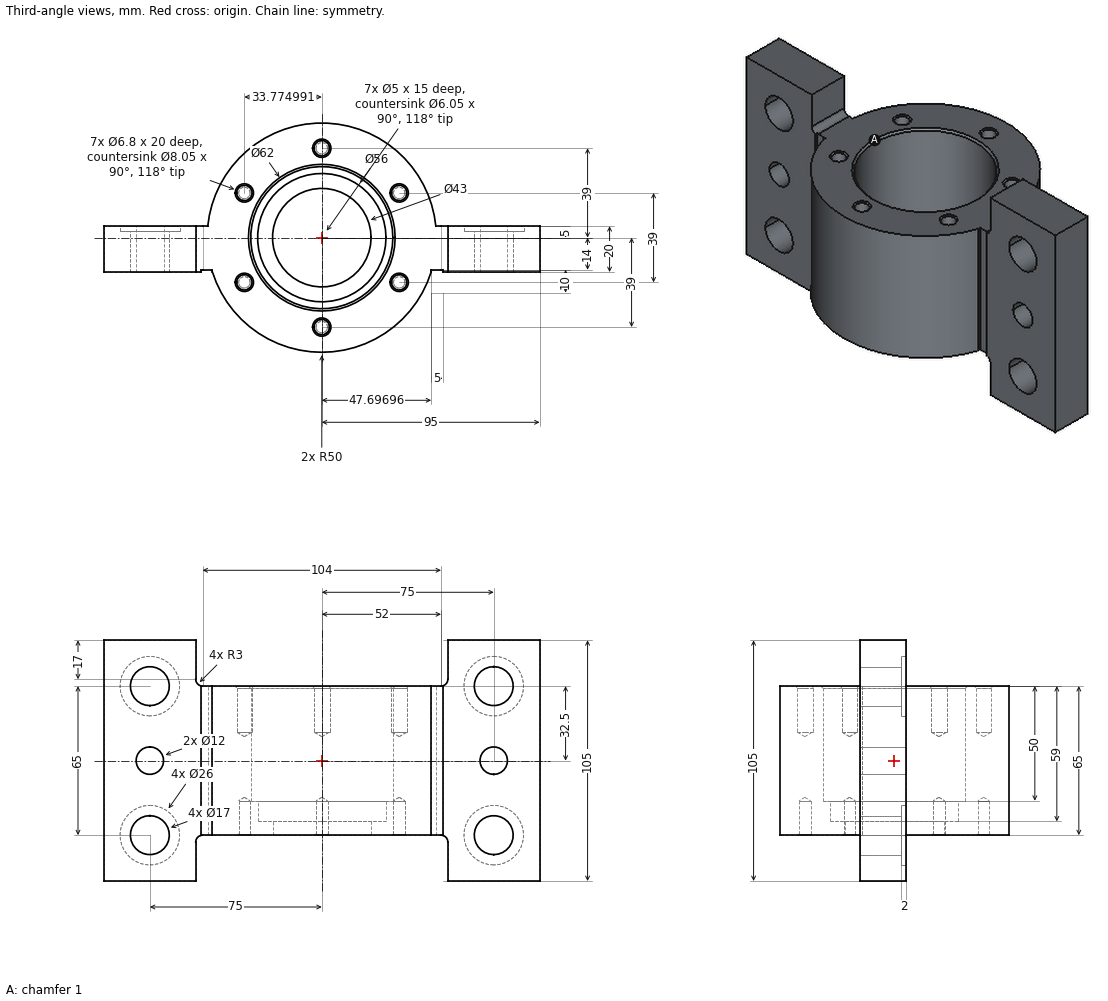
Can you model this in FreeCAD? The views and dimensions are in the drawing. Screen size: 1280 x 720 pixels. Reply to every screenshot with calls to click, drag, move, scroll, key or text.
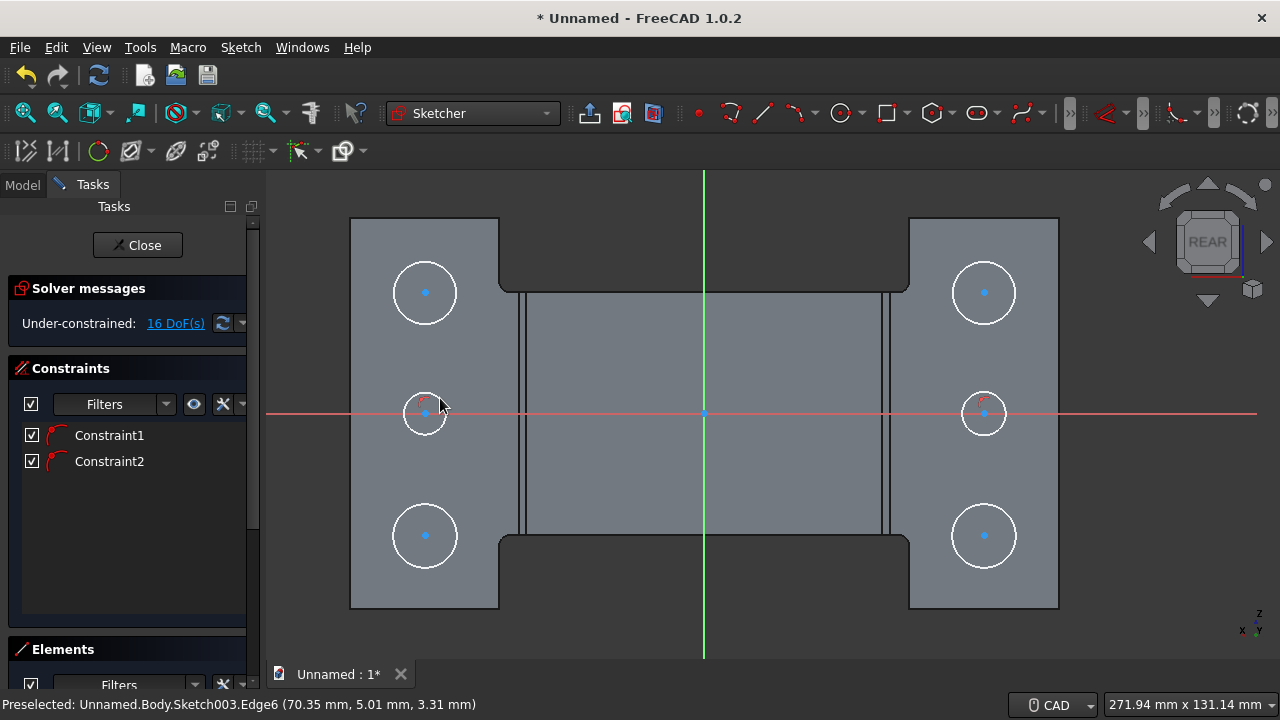
click(1006, 513)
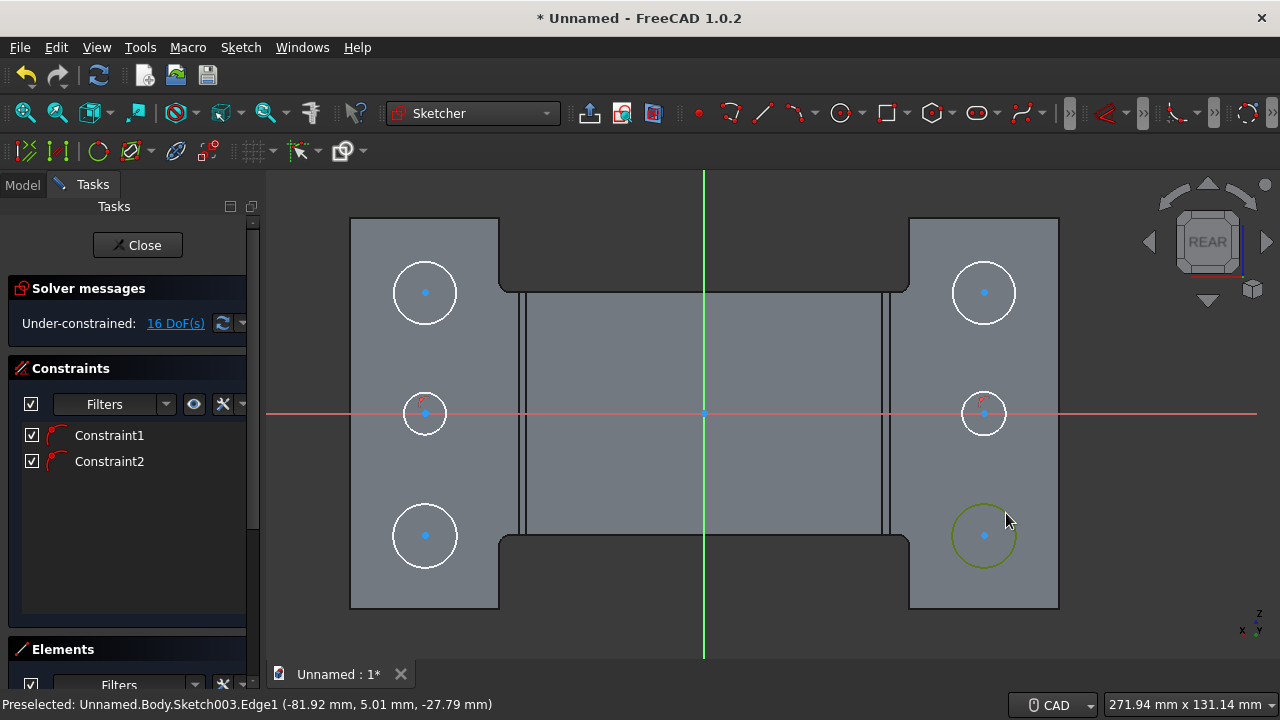
click(1006, 271)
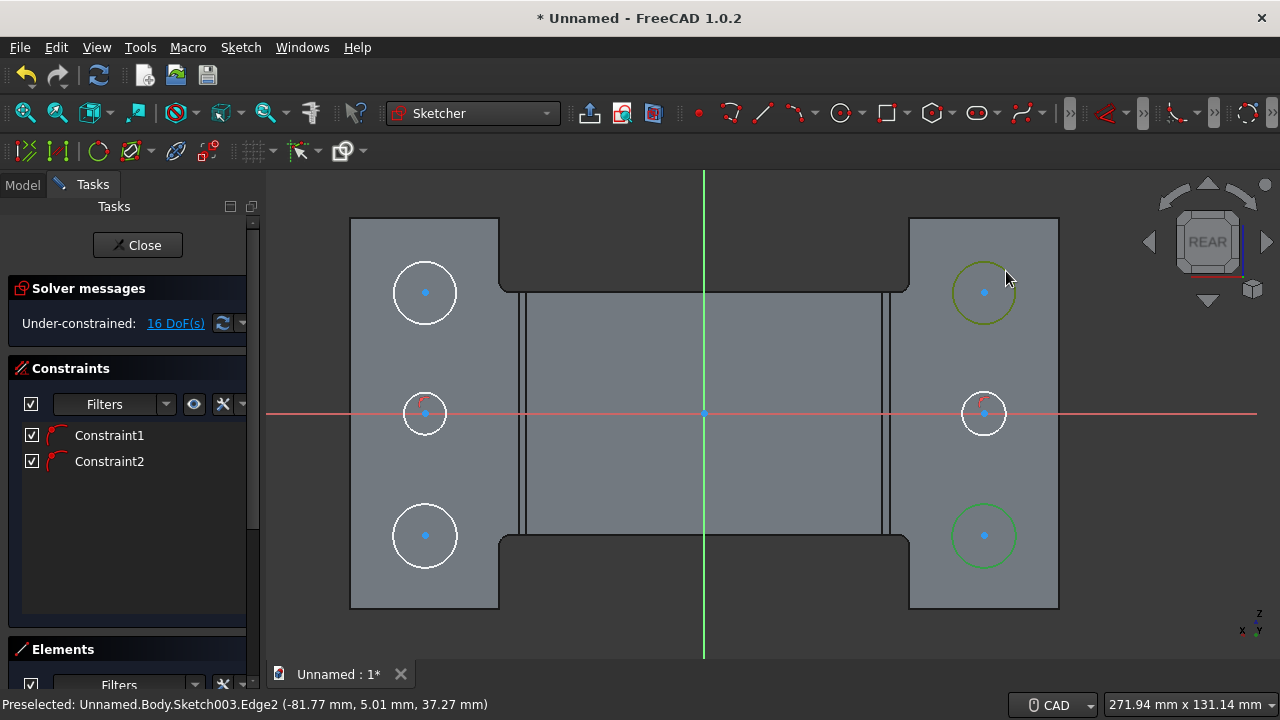
click(447, 271)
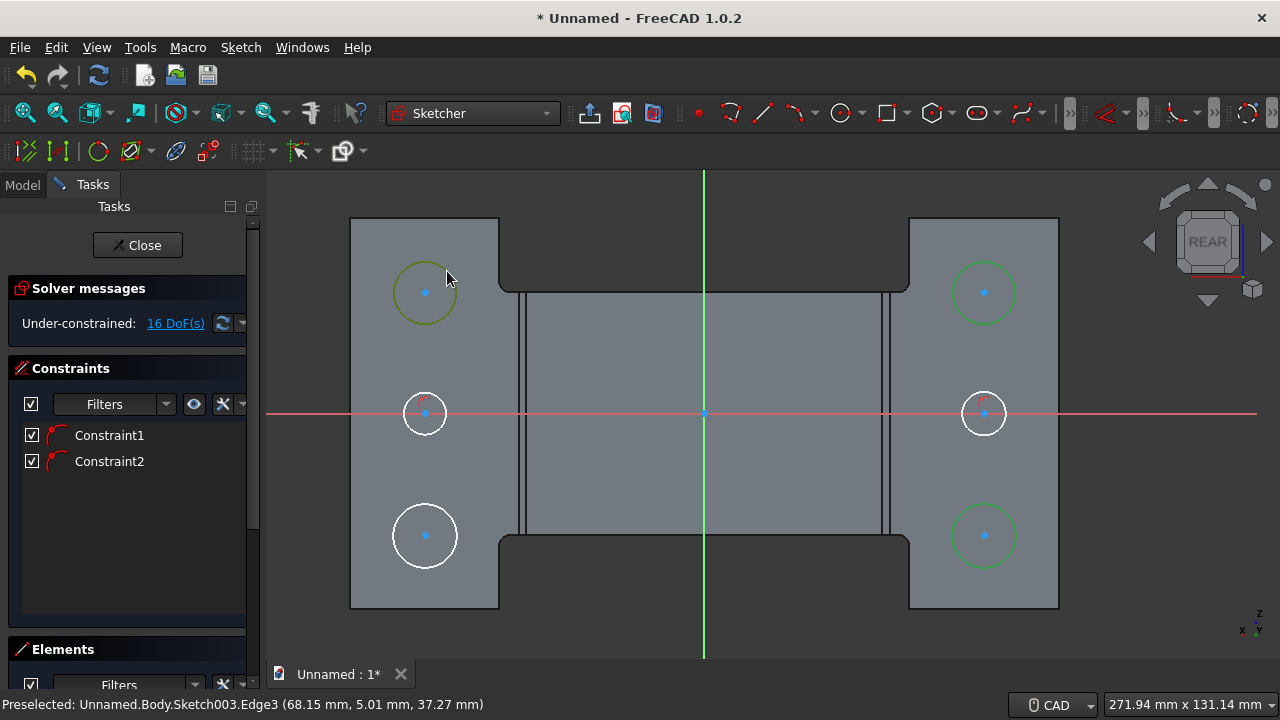
click(447, 513)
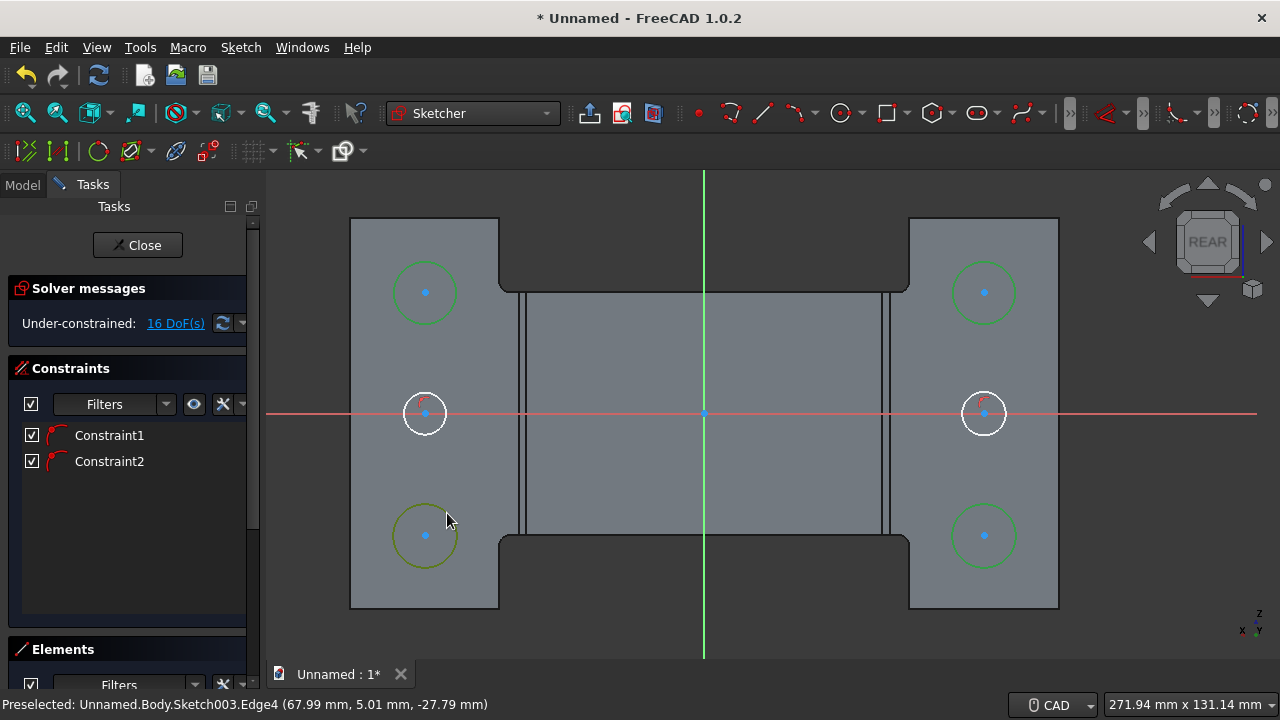
key(e)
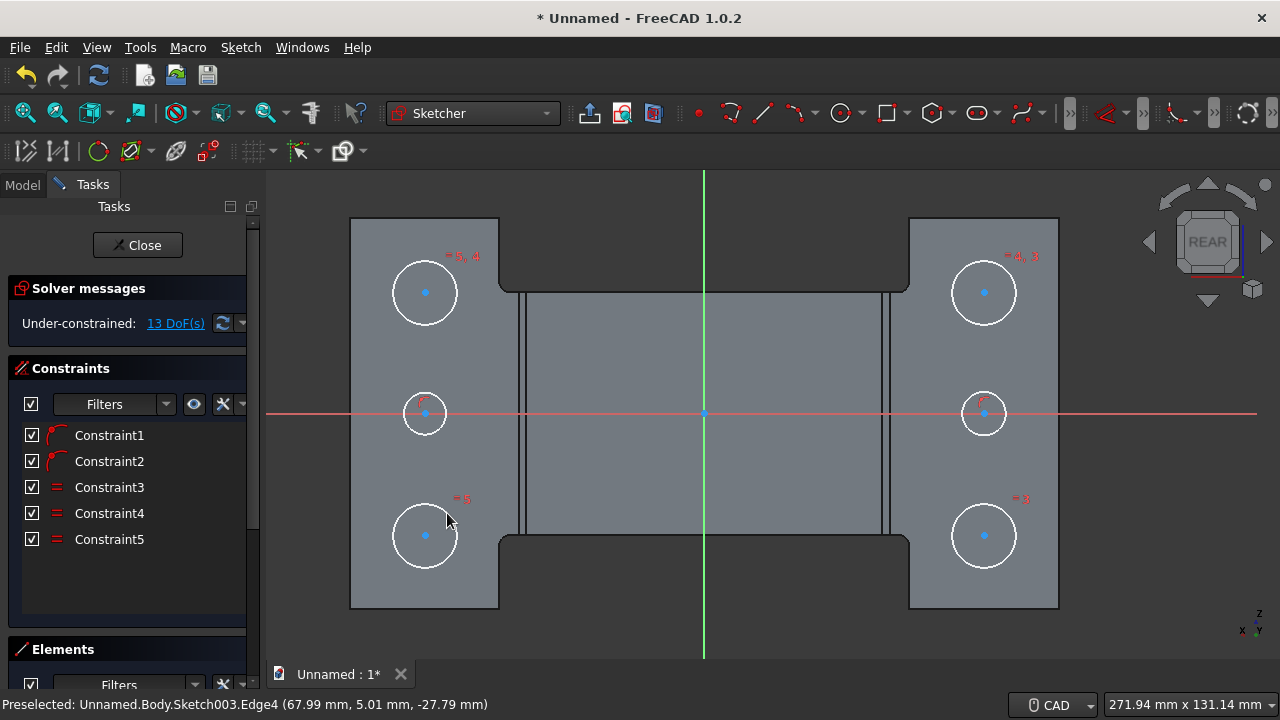
click(999, 398)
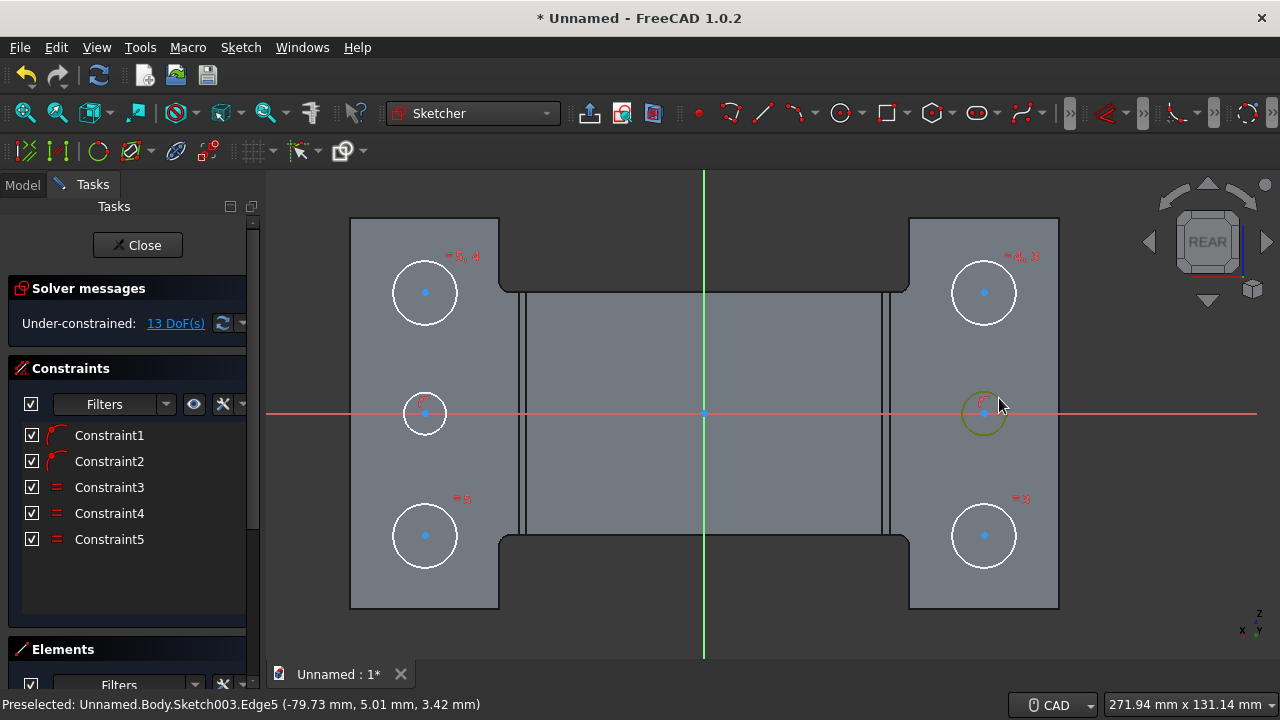
click(440, 399)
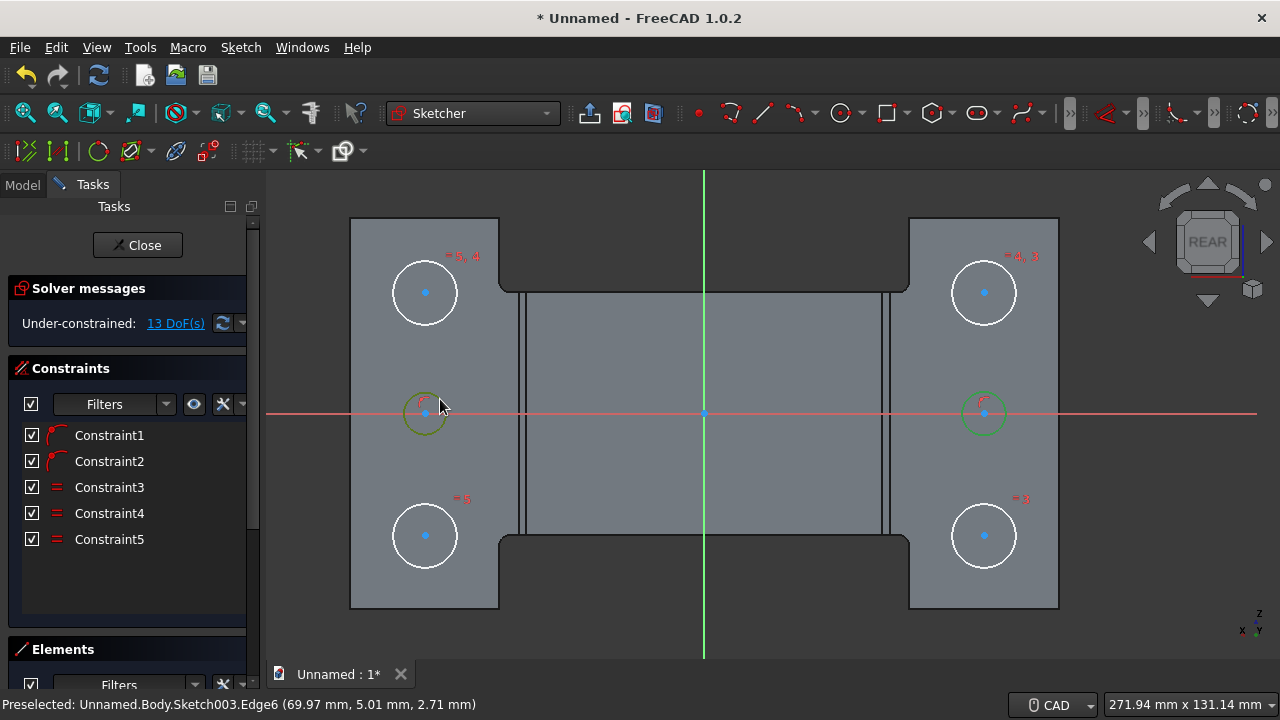
key(e)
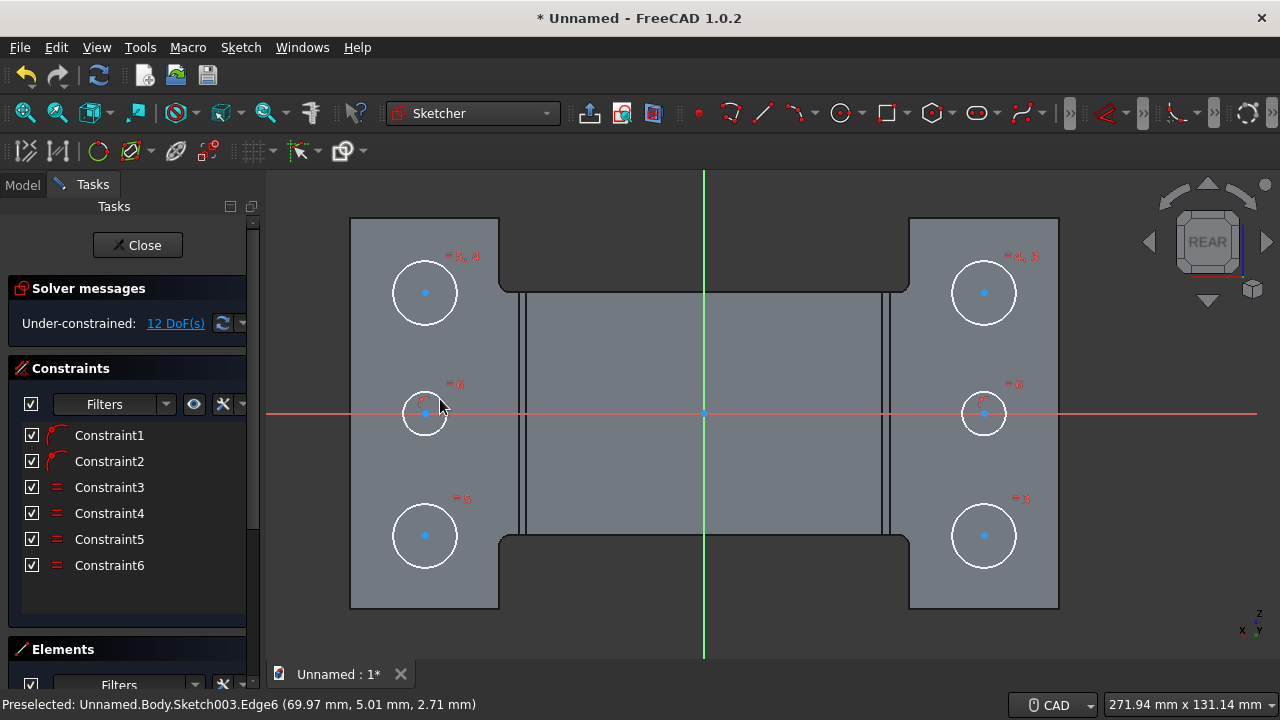
click(984, 536)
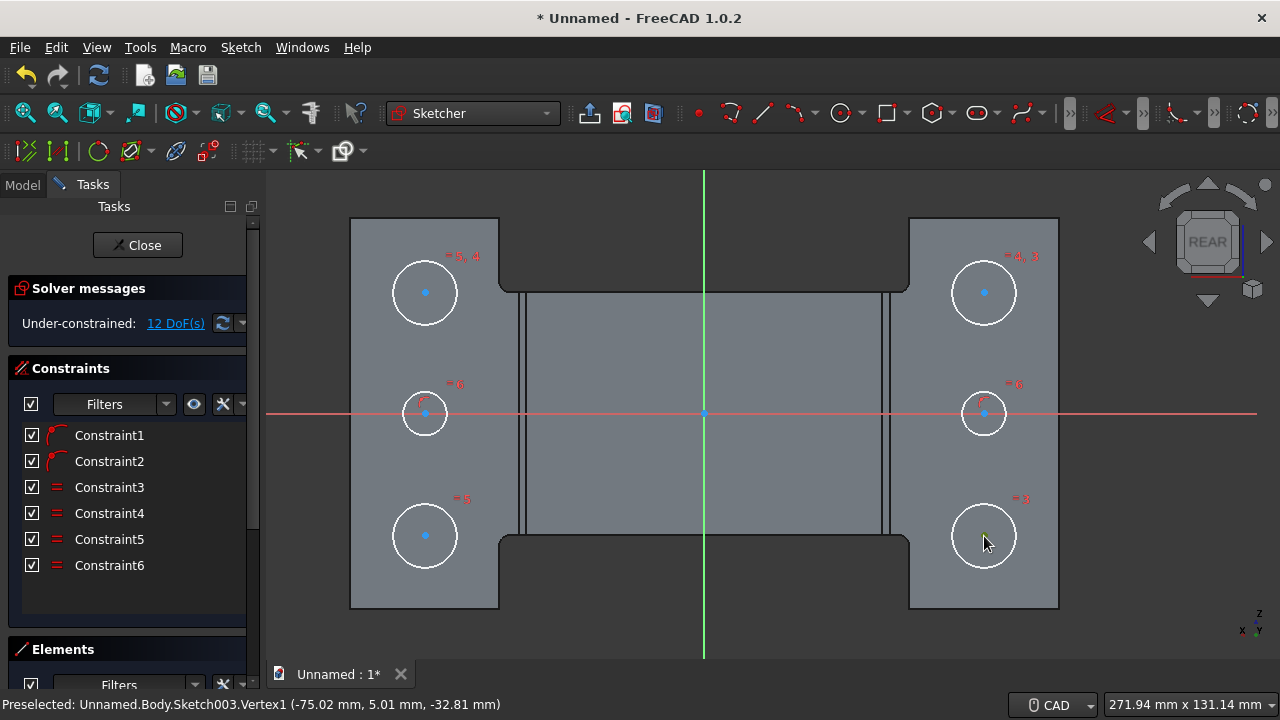
click(984, 293)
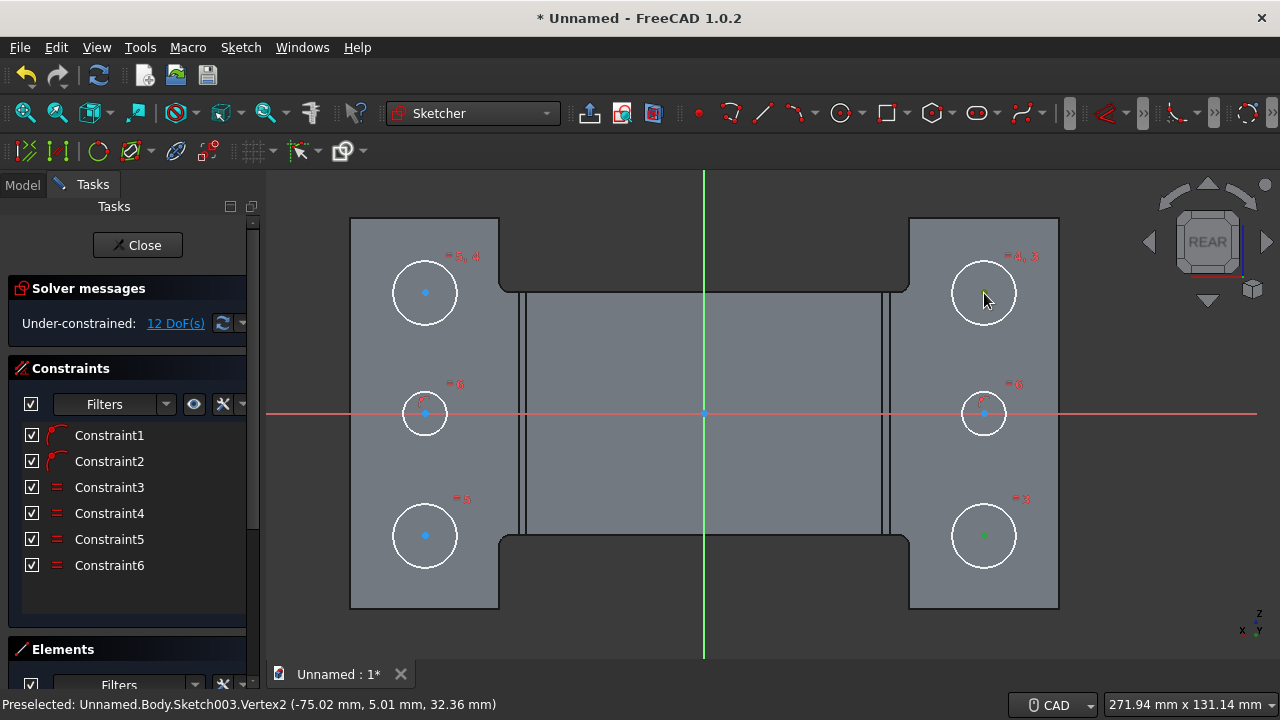
click(353, 414)